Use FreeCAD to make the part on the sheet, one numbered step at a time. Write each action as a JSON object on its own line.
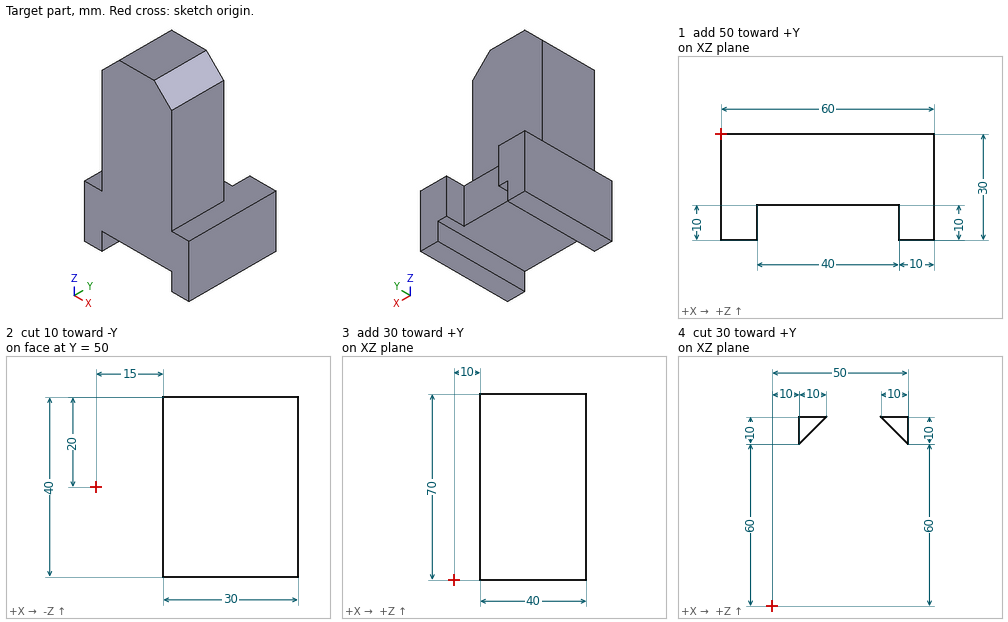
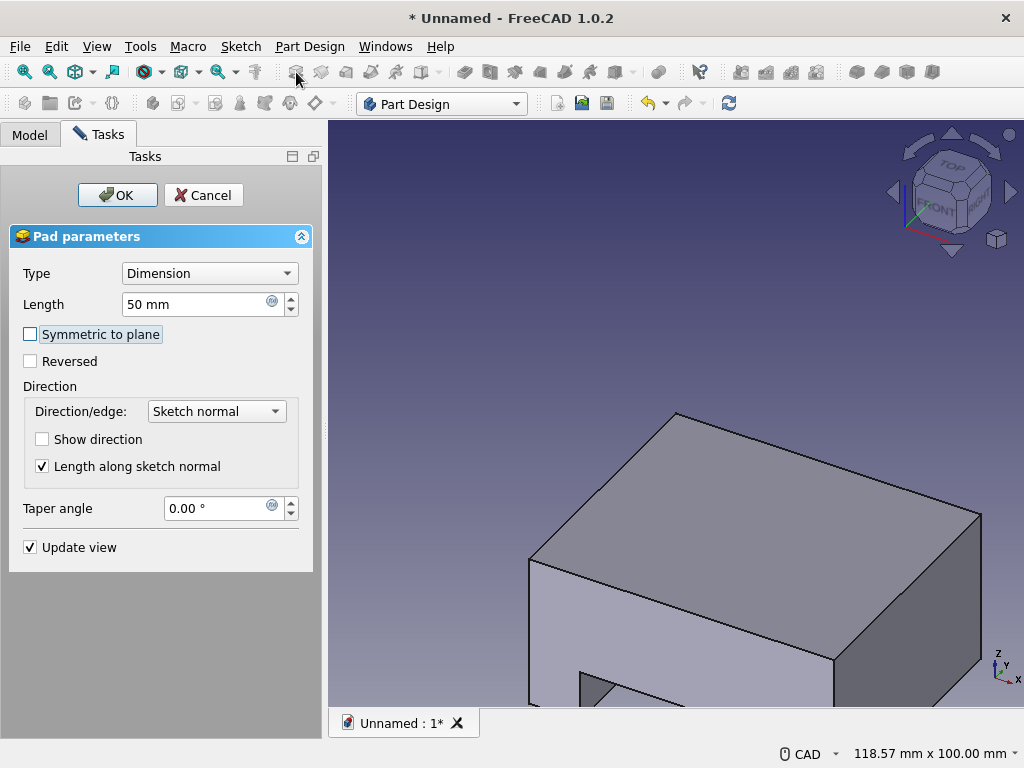
{"action": "left_click", "coordinate": [31, 361]}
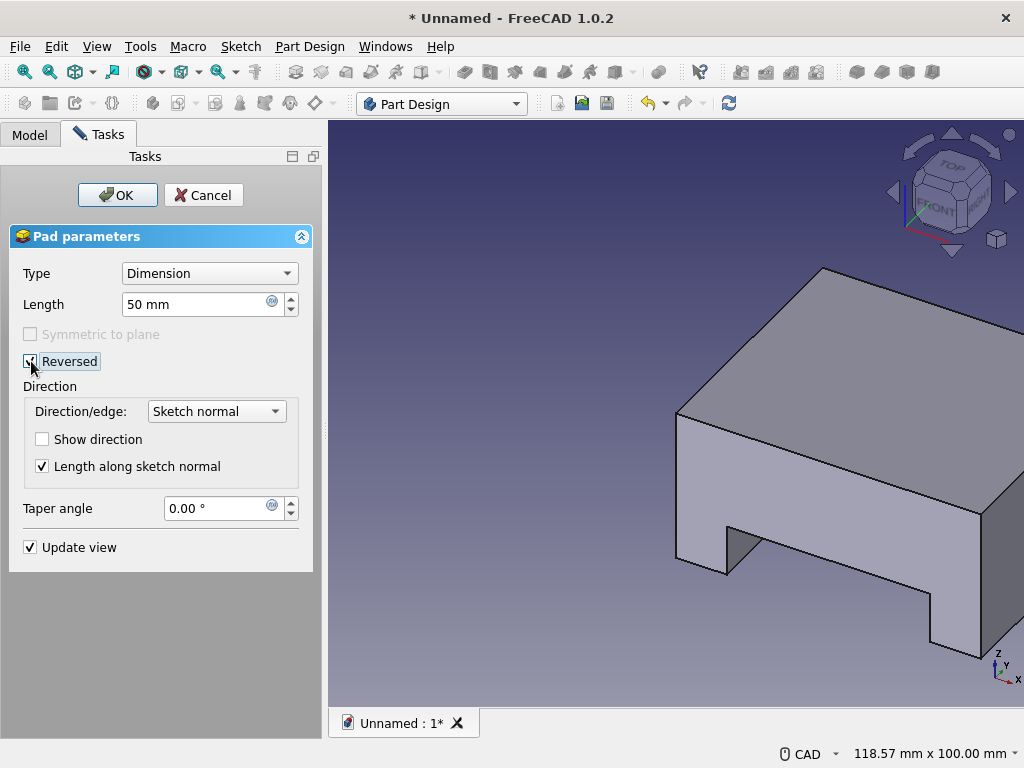
{"action": "left_click", "coordinate": [118, 195]}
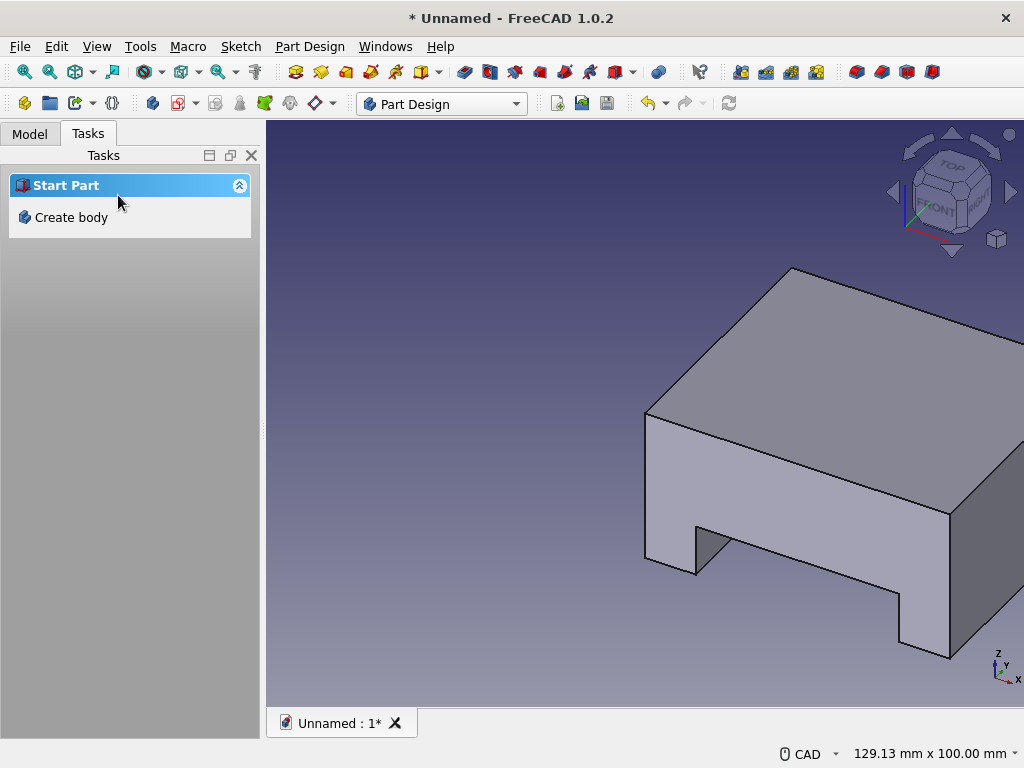
{"action": "left_click", "coordinate": [25, 72]}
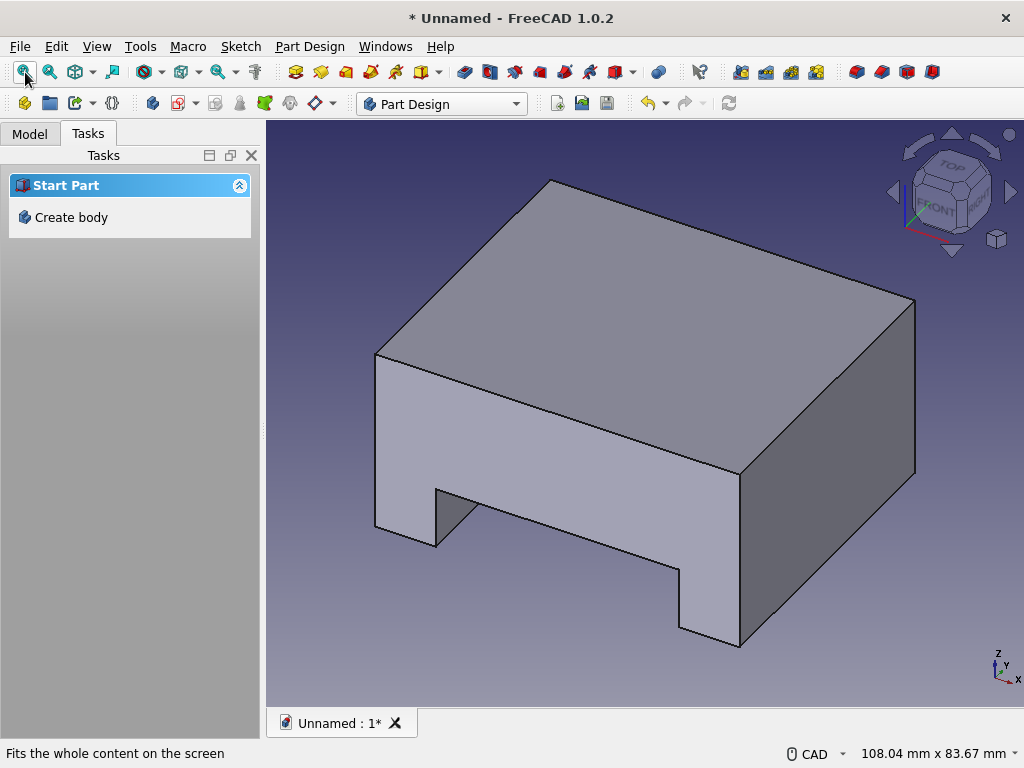
{"action": "key", "text": "4"}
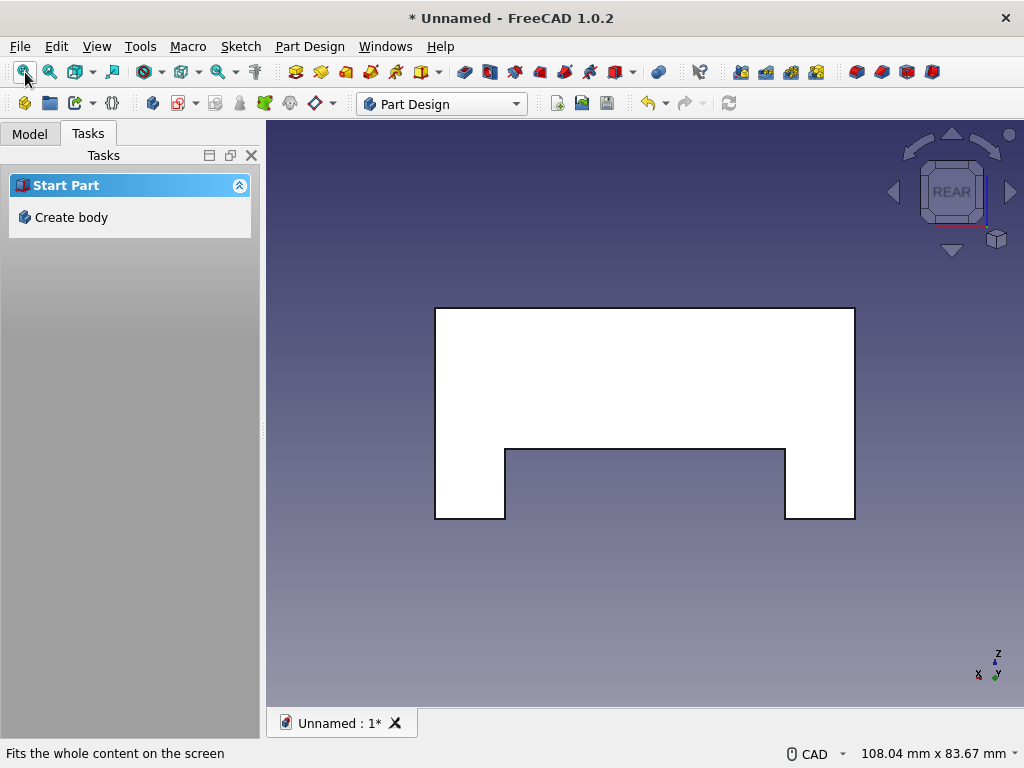
{"action": "left_click", "coordinate": [525, 382]}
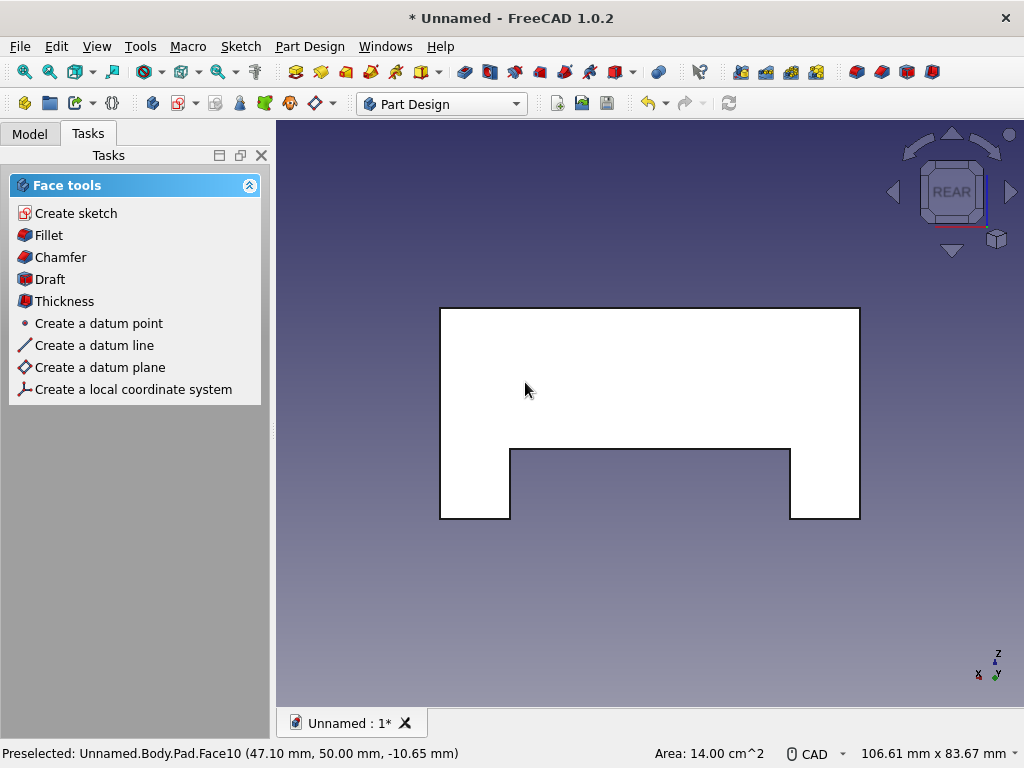
{"action": "left_click", "coordinate": [178, 104]}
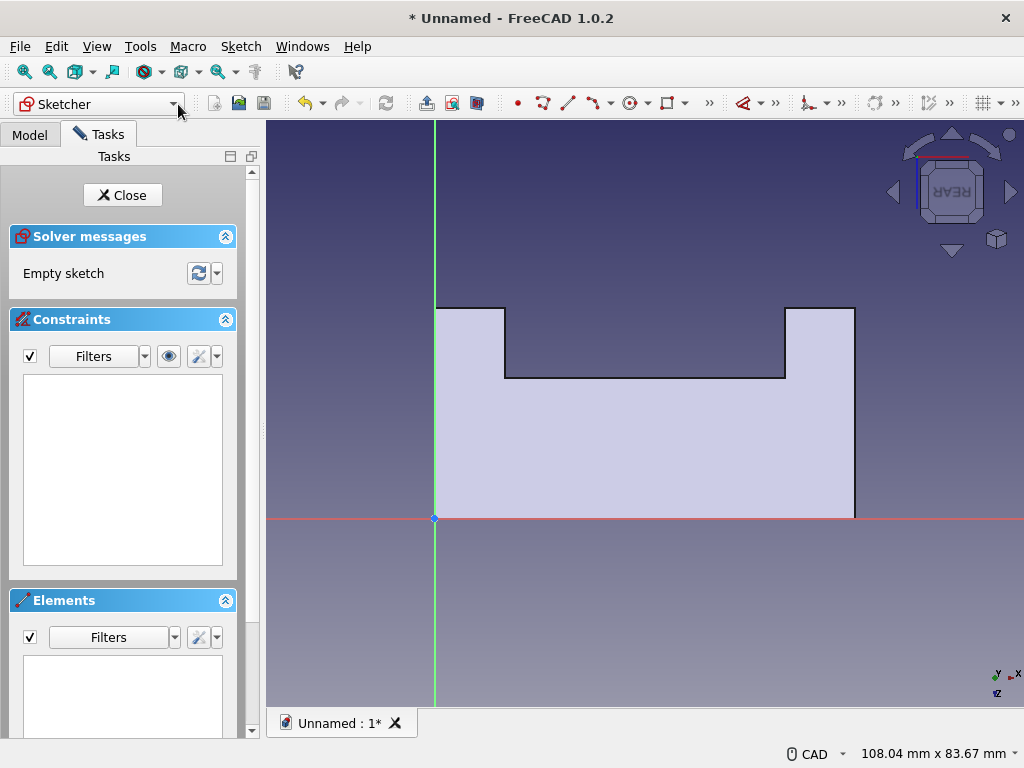
{"action": "scroll", "coordinate": [505, 148], "scroll_direction": "down", "scroll_amount": 1}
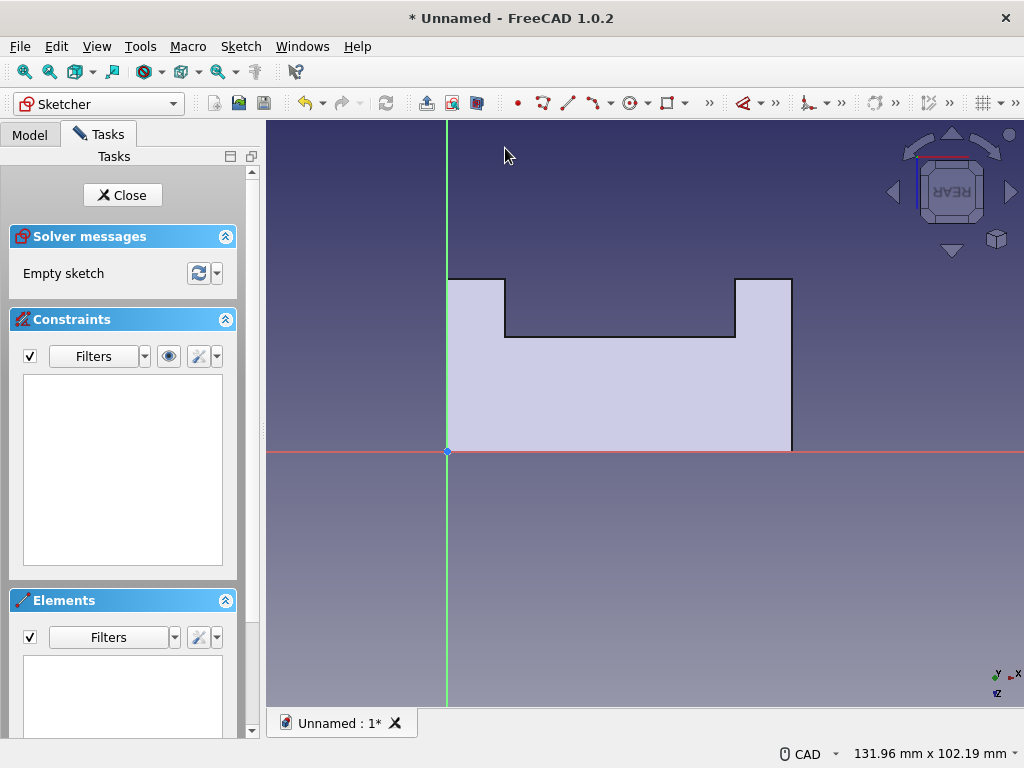
{"action": "scroll", "coordinate": [577, 529], "scroll_direction": "up", "scroll_amount": 2}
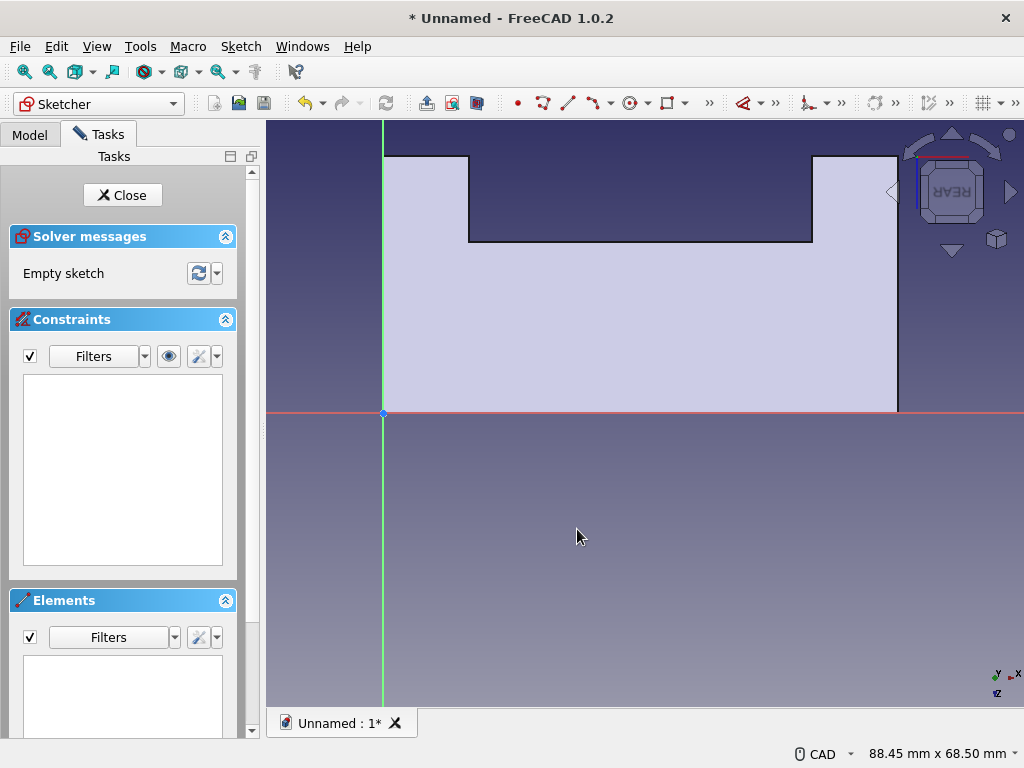
{"action": "left_click", "coordinate": [666, 104]}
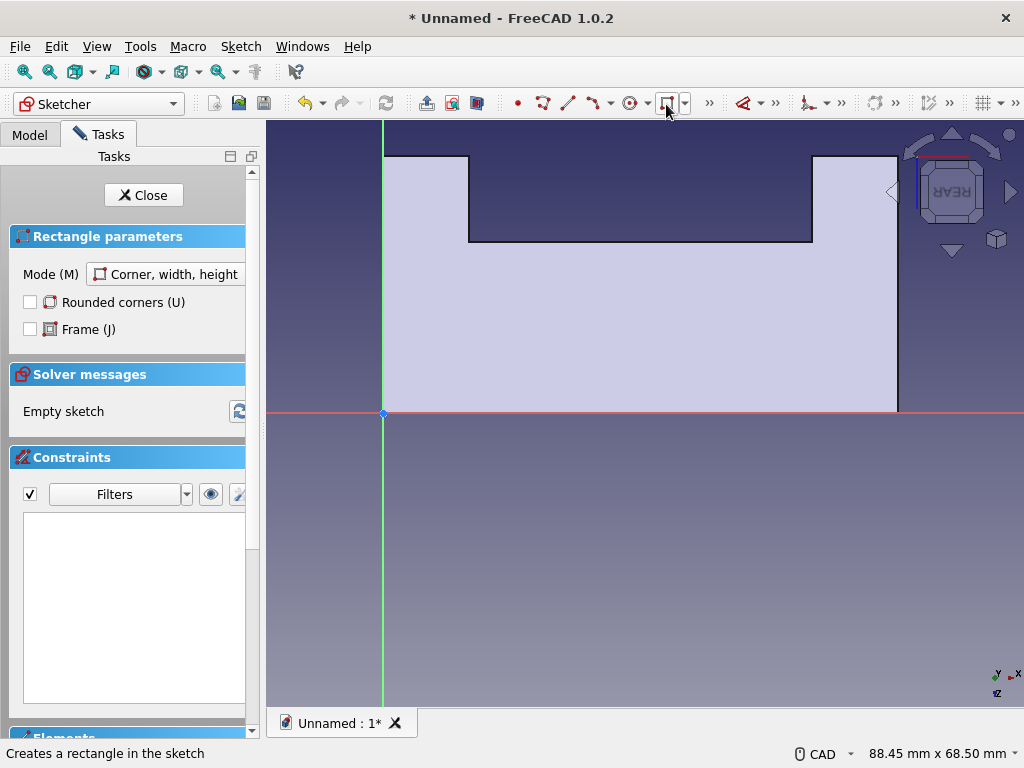
{"action": "left_click", "coordinate": [512, 242]}
{"action": "left_click", "coordinate": [769, 584]}
{"action": "key", "text": "Escape"}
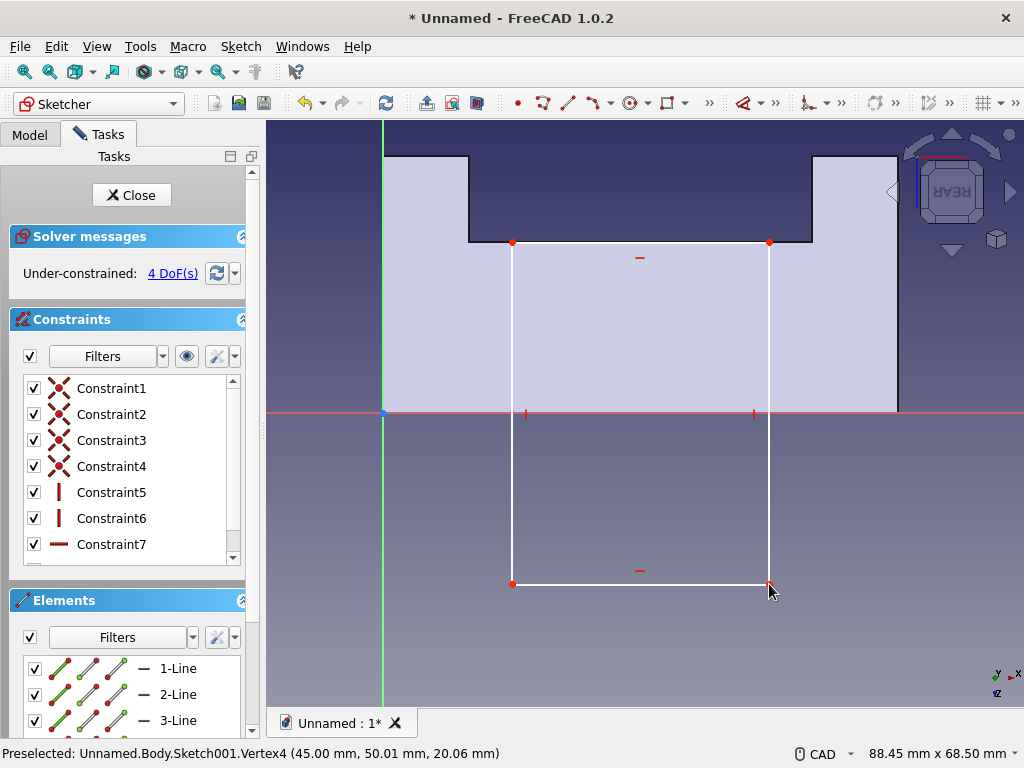
{"action": "left_click", "coordinate": [742, 104]}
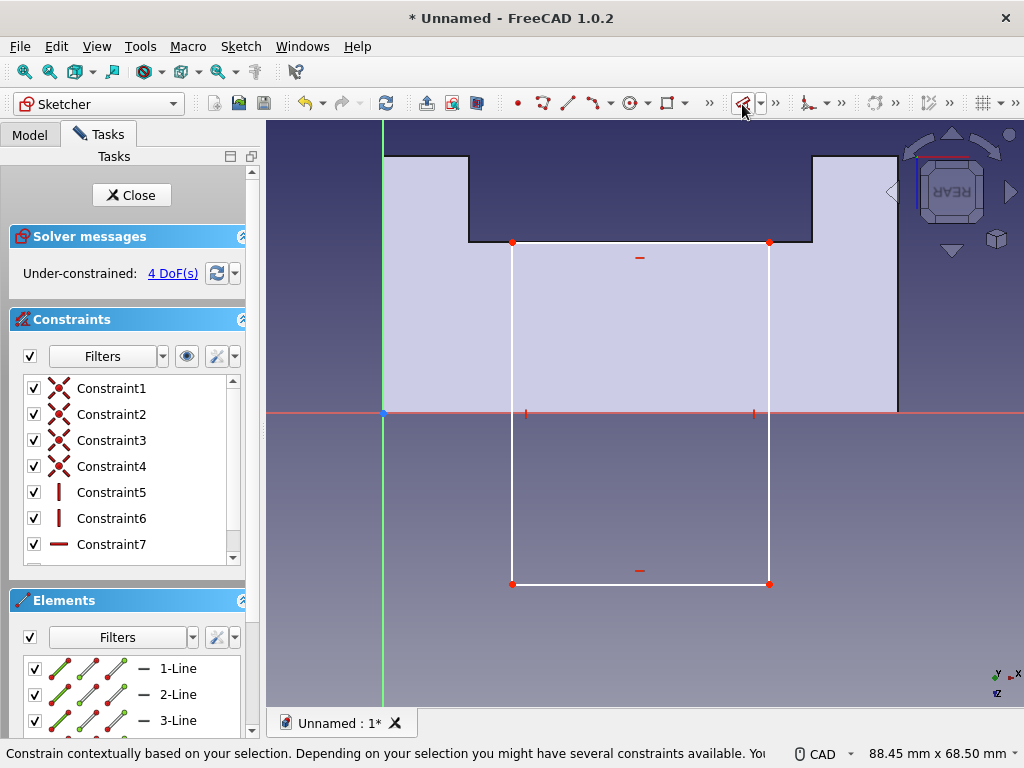
{"action": "left_click", "coordinate": [512, 346]}
{"action": "left_click", "coordinate": [478, 335]}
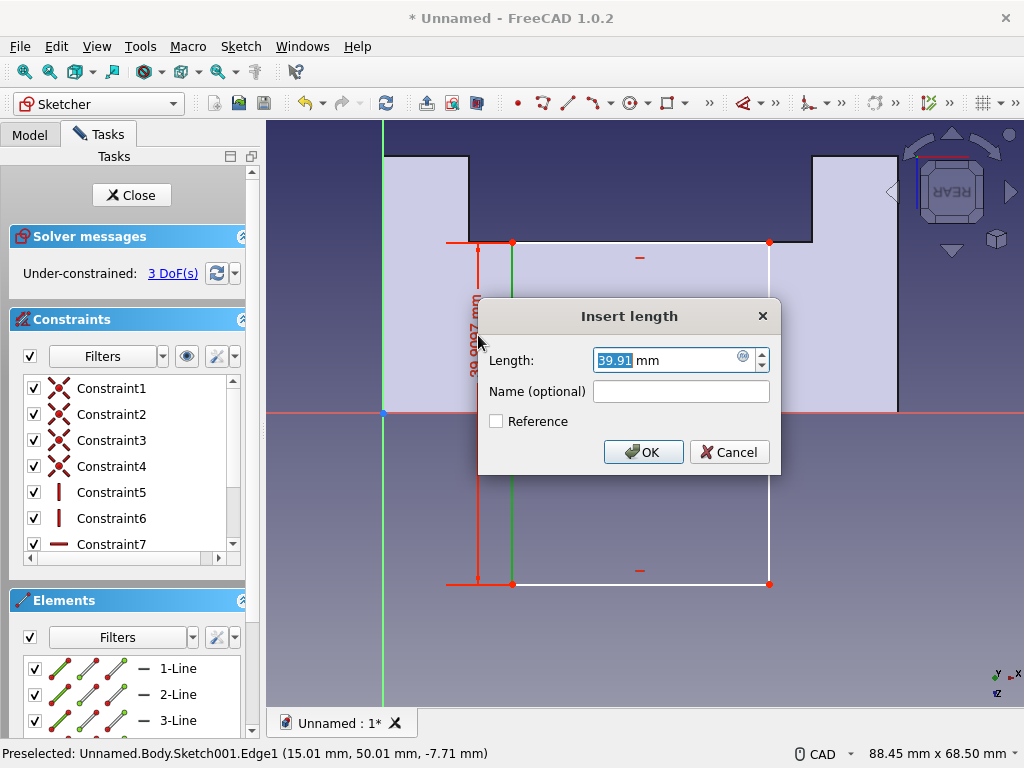
{"action": "type", "text": "40"}
{"action": "key", "text": "Return"}